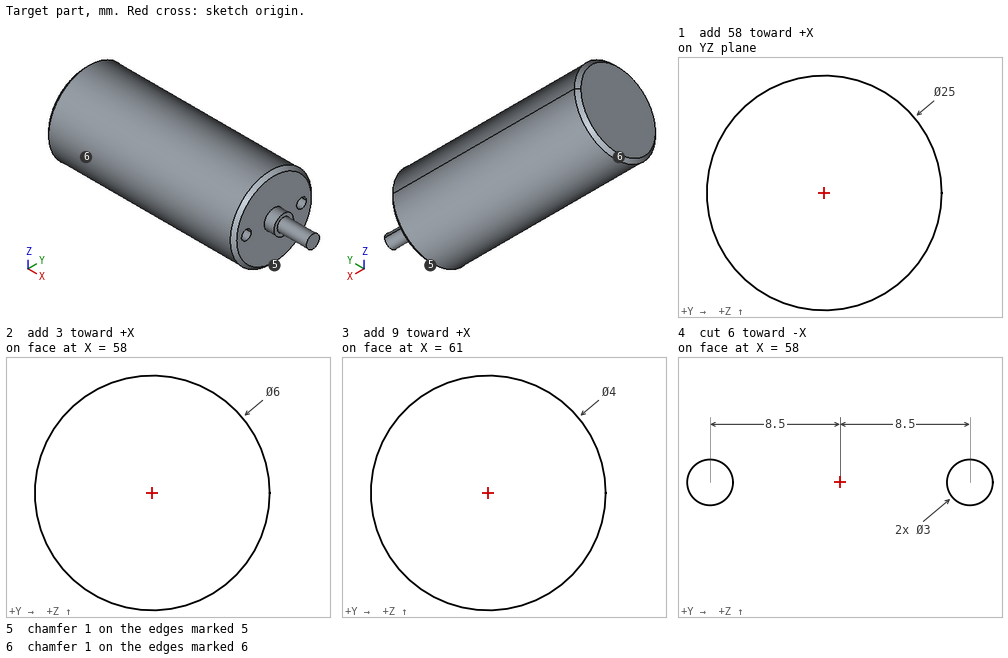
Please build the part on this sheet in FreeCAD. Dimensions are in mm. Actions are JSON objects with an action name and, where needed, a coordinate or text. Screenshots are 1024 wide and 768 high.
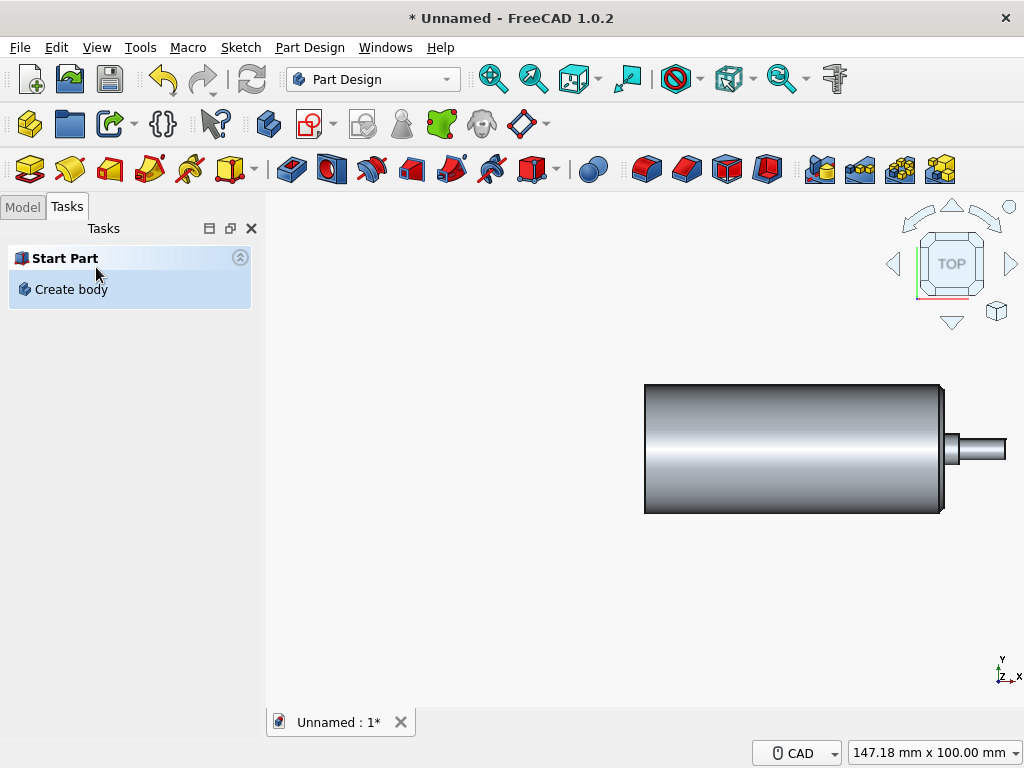
{"action": "left_click", "coordinate": [645, 501]}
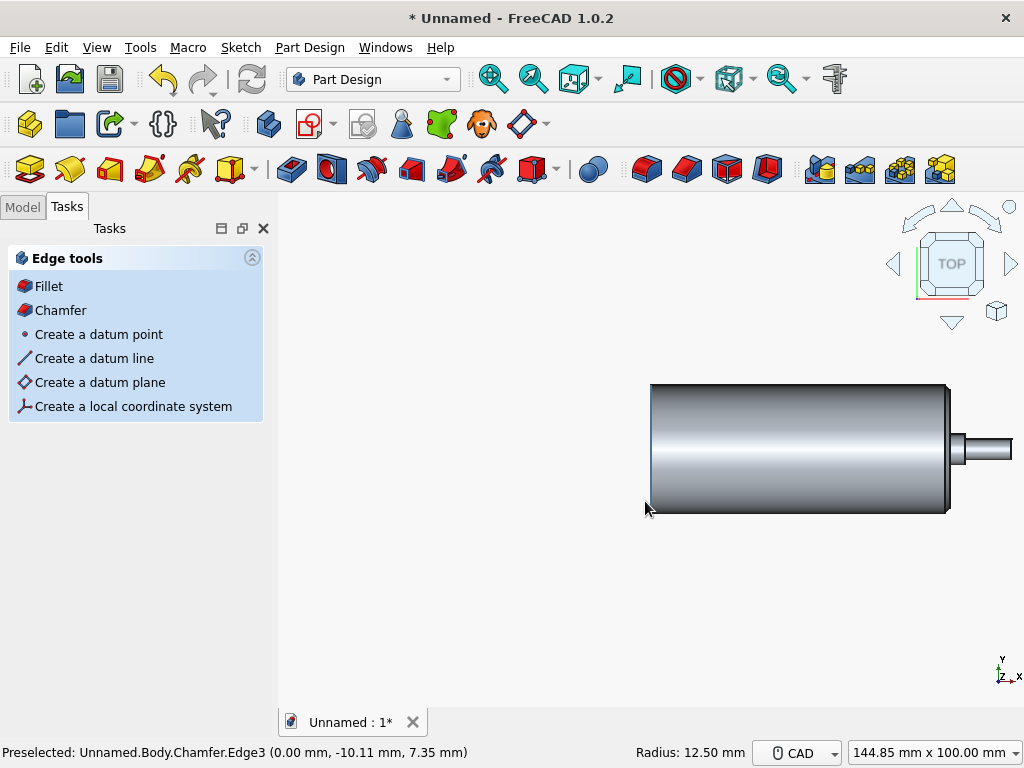
{"action": "left_click", "coordinate": [688, 170]}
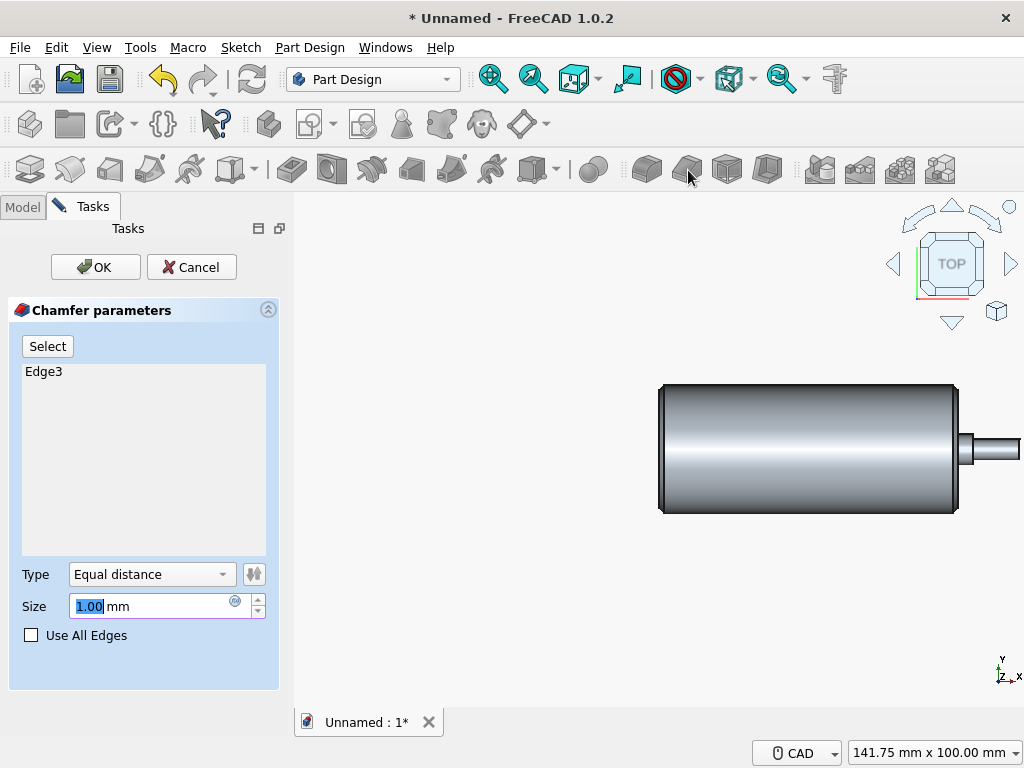
{"action": "type", "text": "1"}
{"action": "key", "text": "Tab"}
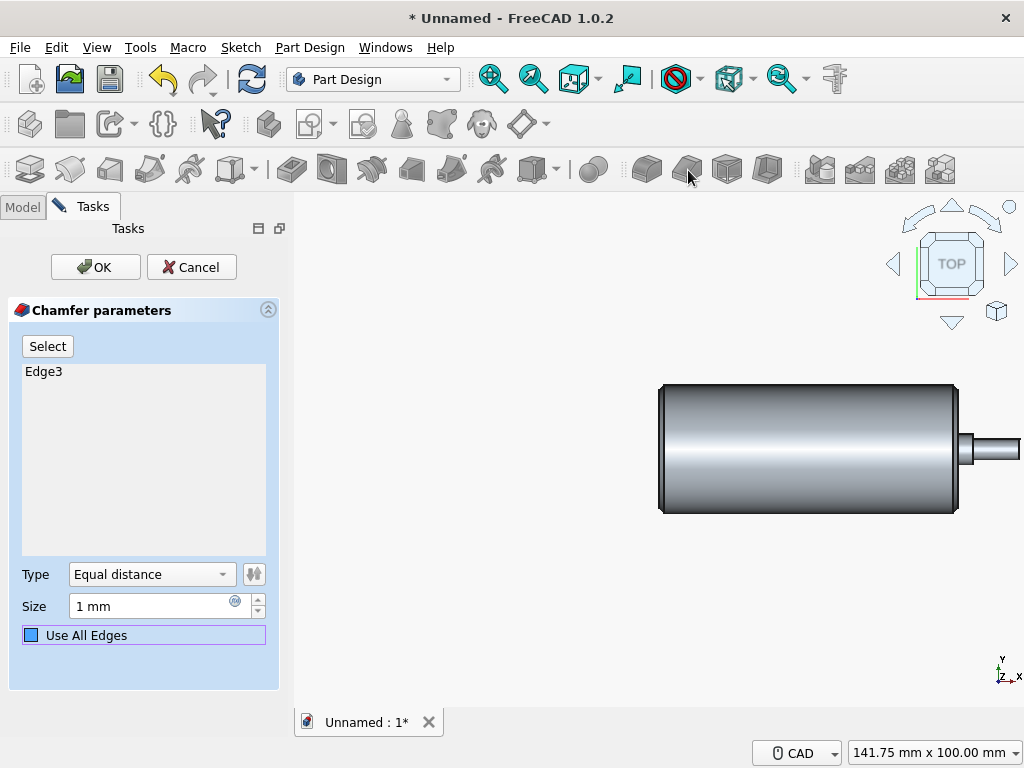
{"action": "left_click", "coordinate": [96, 267]}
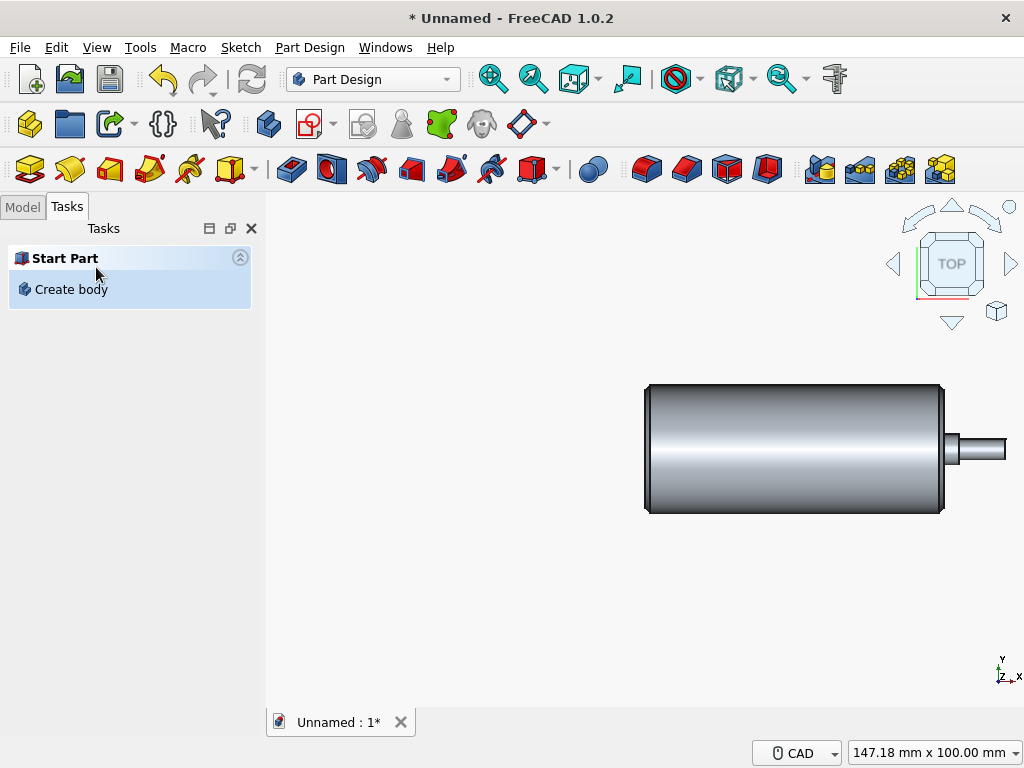
{"action": "key", "text": "0"}